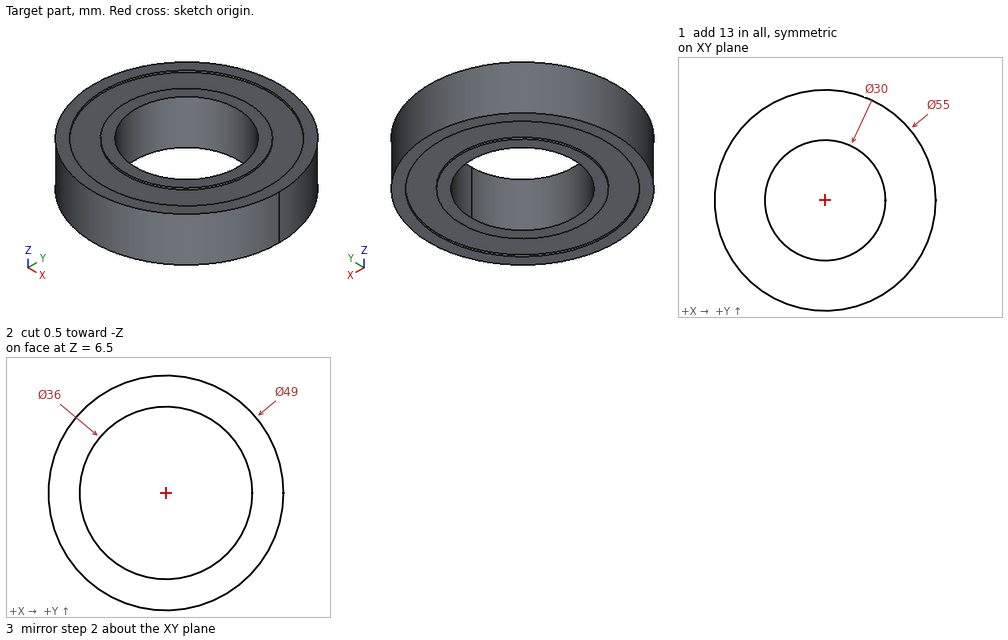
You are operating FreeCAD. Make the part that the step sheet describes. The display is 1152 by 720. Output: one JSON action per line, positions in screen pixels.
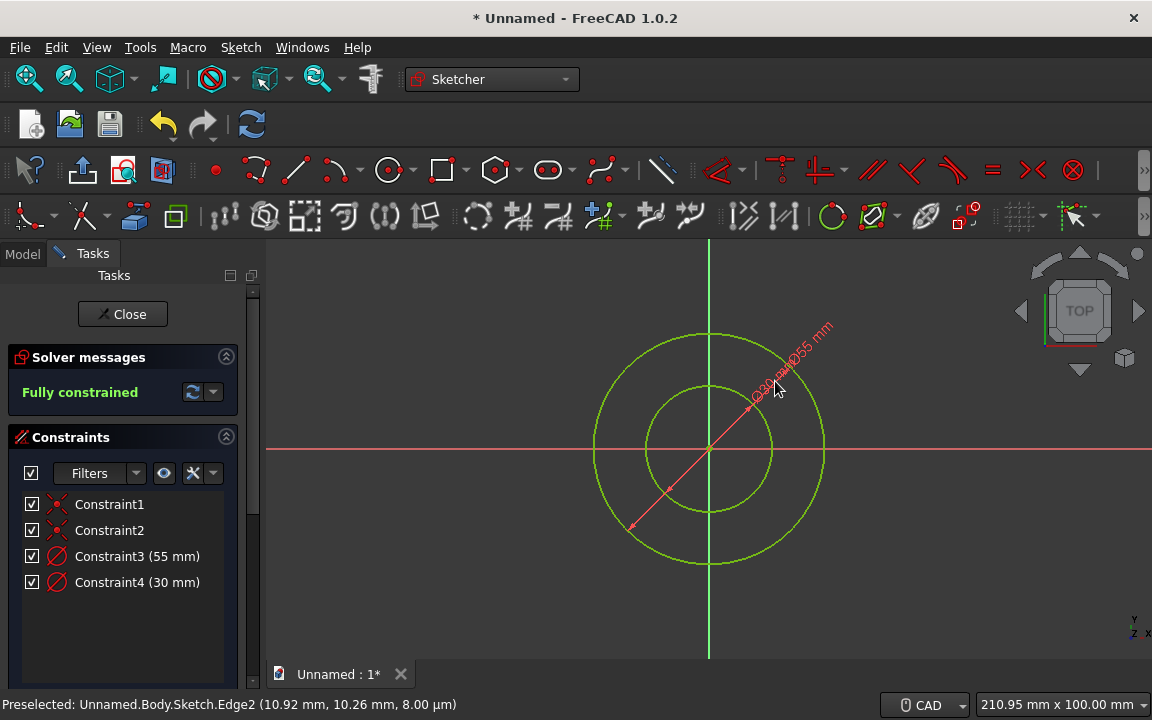
{"action": "left_click", "coordinate": [123, 314]}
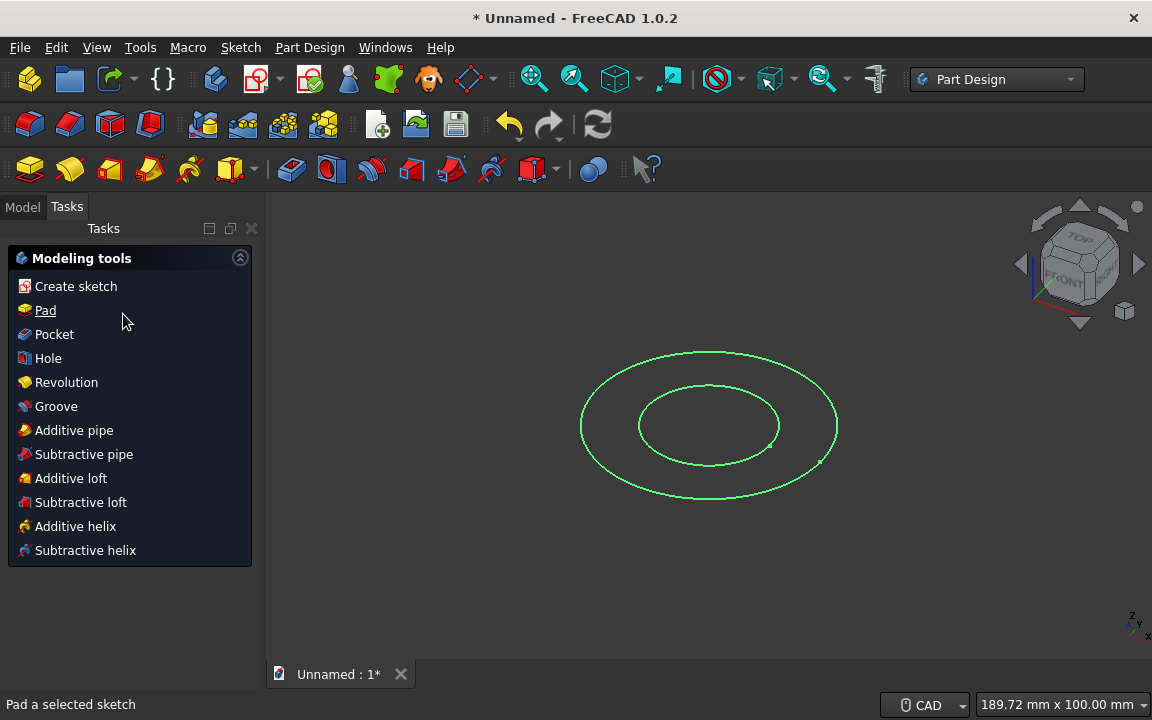
{"action": "left_click", "coordinate": [30, 170]}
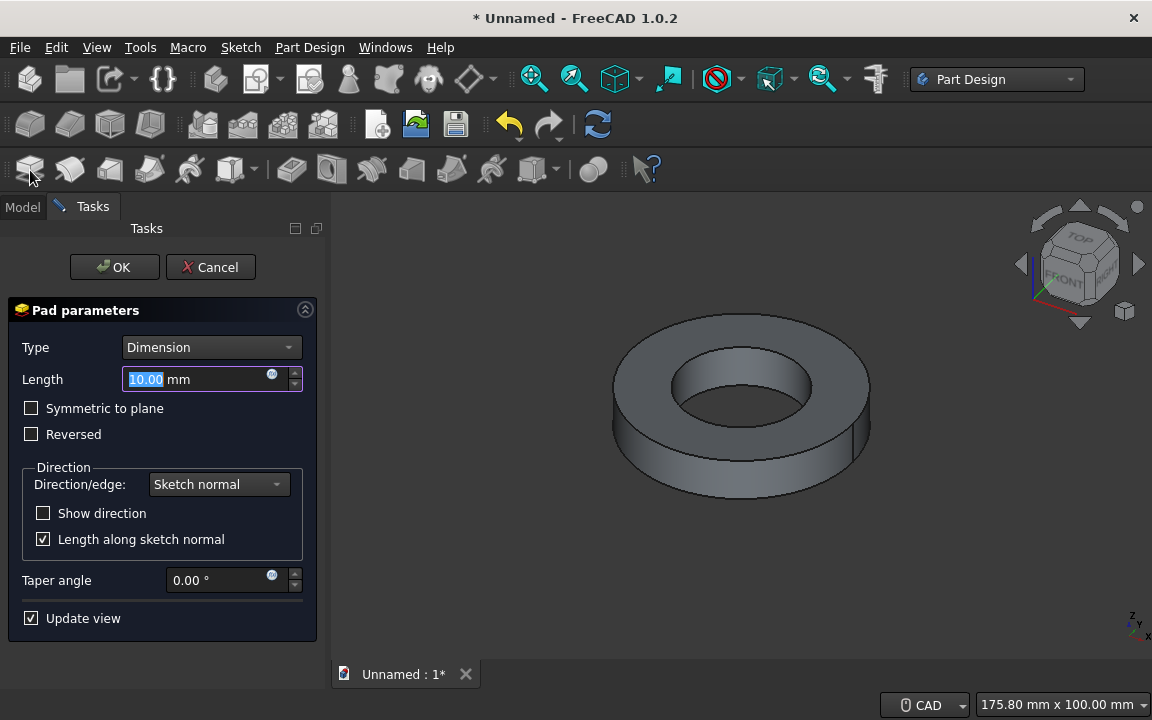
{"action": "type", "text": "13"}
{"action": "key", "text": "Tab"}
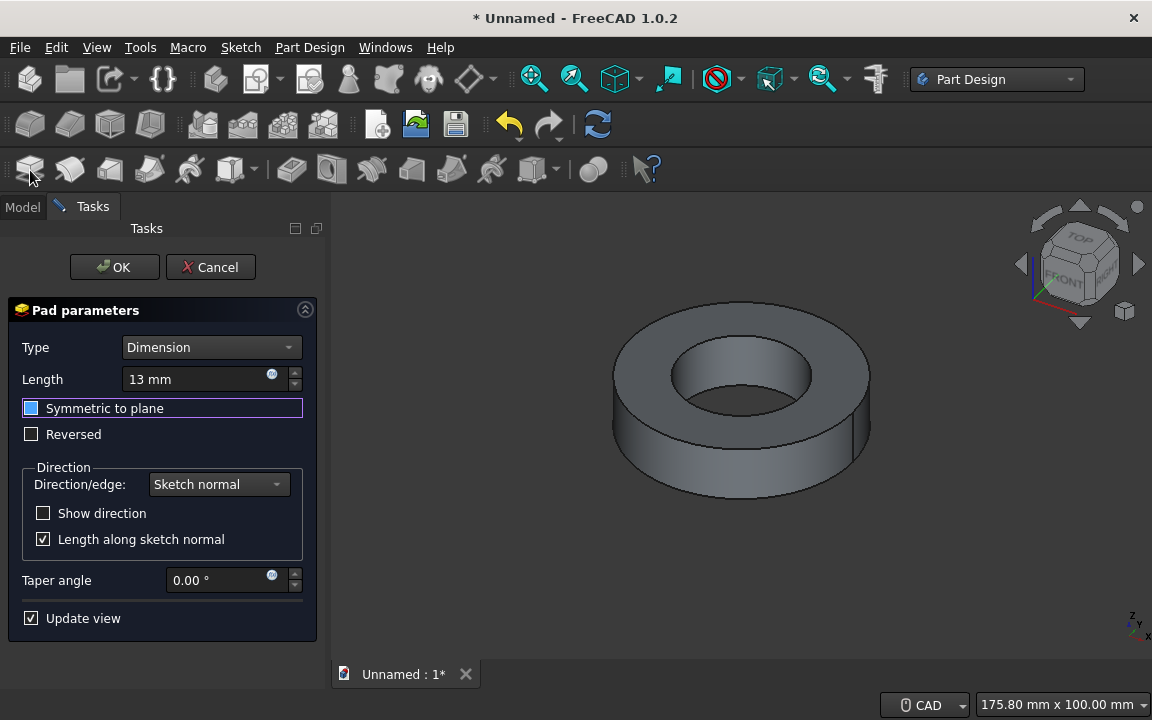
{"action": "left_click", "coordinate": [30, 408]}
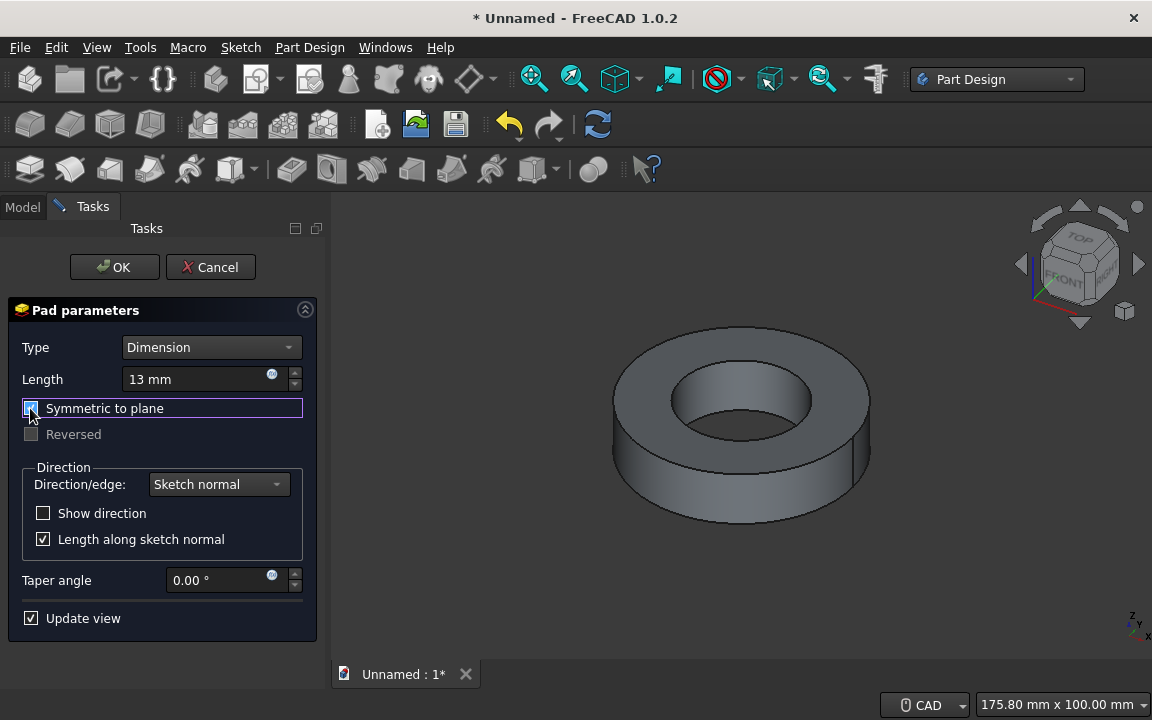
{"action": "left_click", "coordinate": [115, 267]}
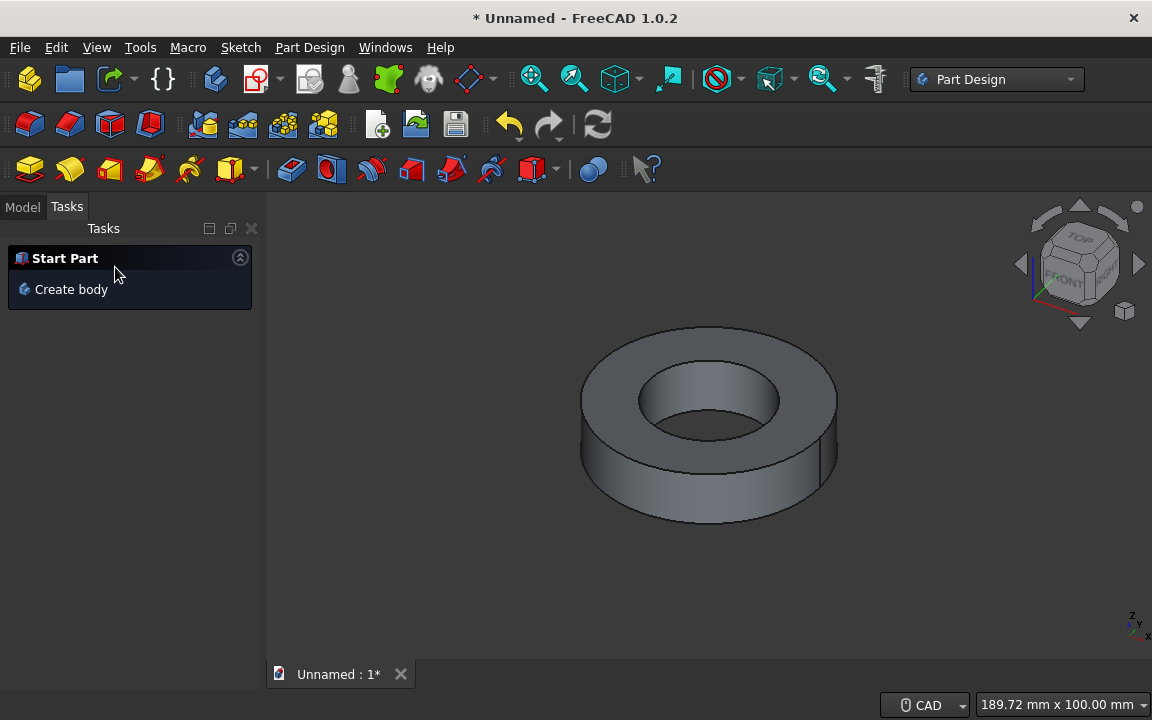
{"action": "left_click", "coordinate": [609, 415]}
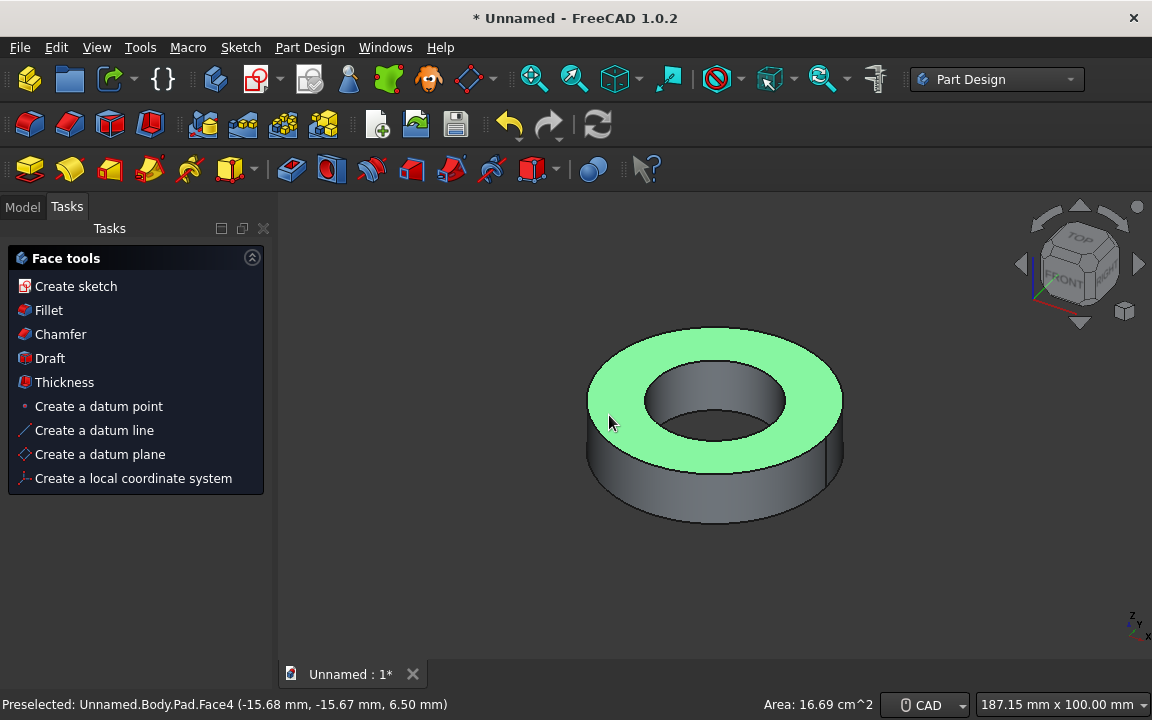
{"action": "left_click", "coordinate": [256, 80]}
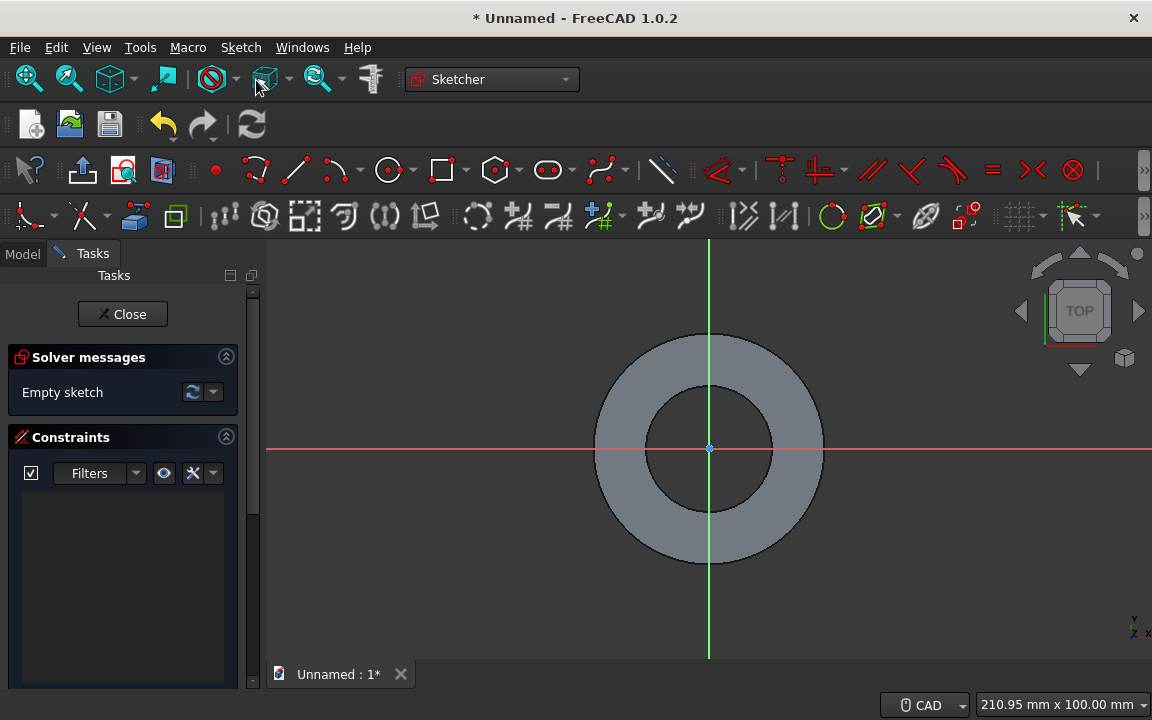
{"action": "left_click", "coordinate": [390, 170]}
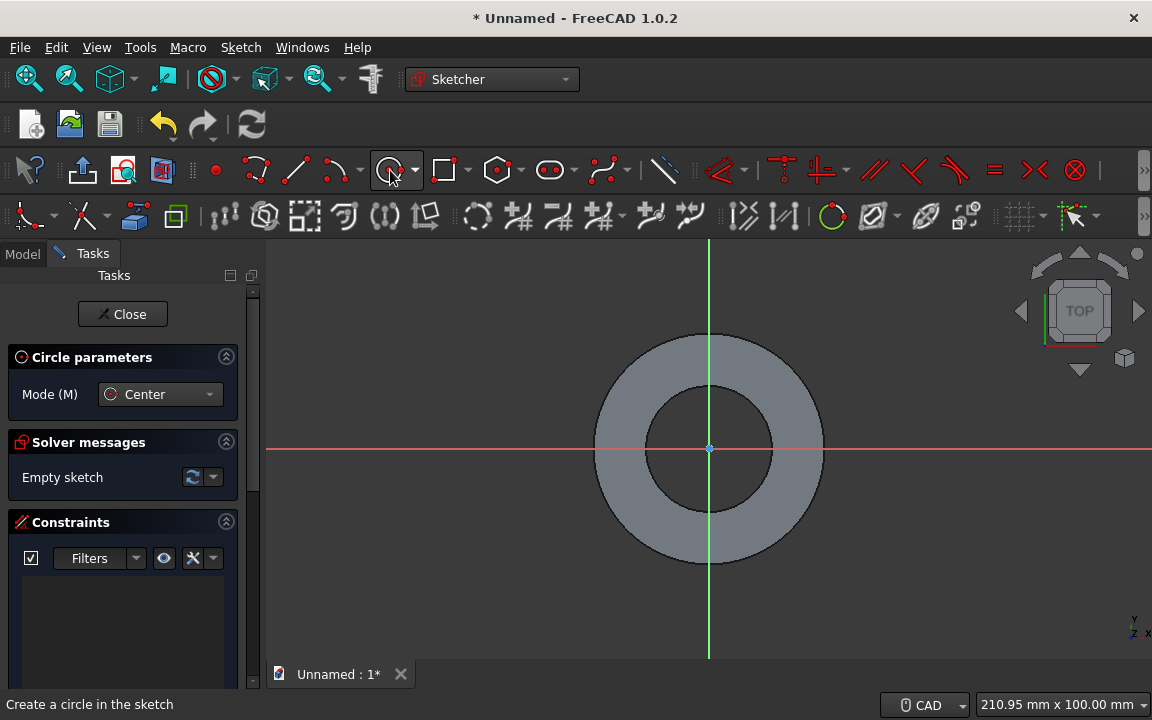
{"action": "left_click", "coordinate": [709, 449]}
{"action": "left_click", "coordinate": [782, 376]}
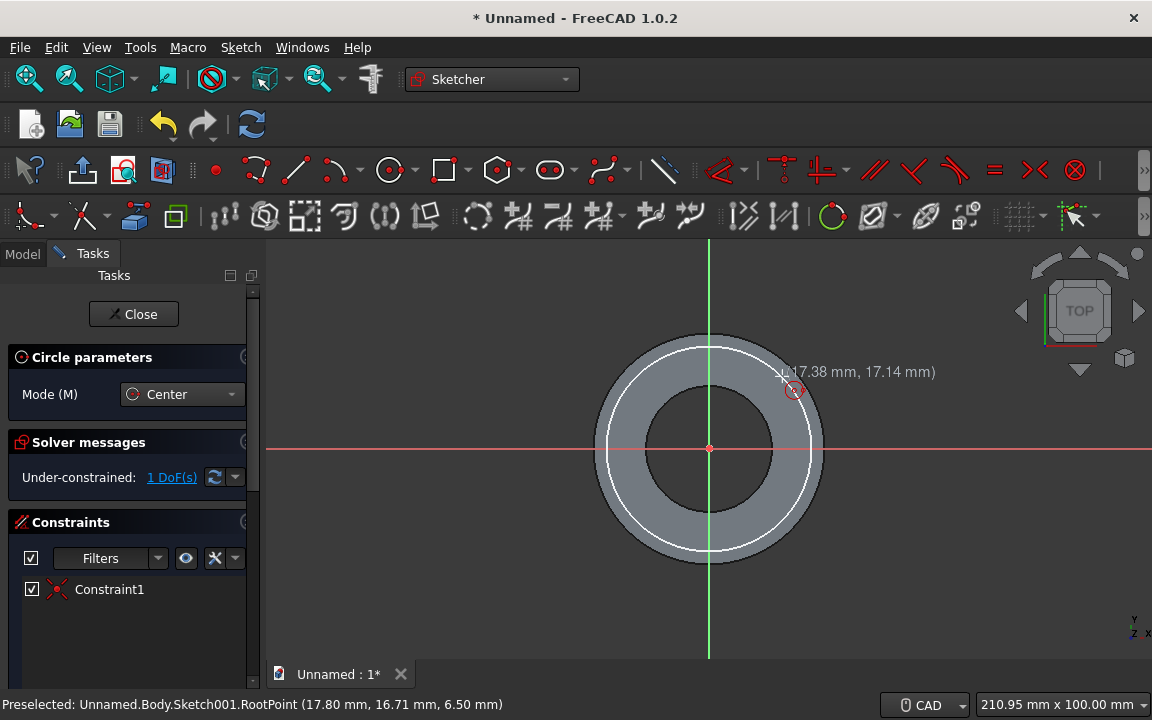
{"action": "left_click", "coordinate": [709, 449]}
{"action": "left_click", "coordinate": [762, 396]}
{"action": "key", "text": "Escape"}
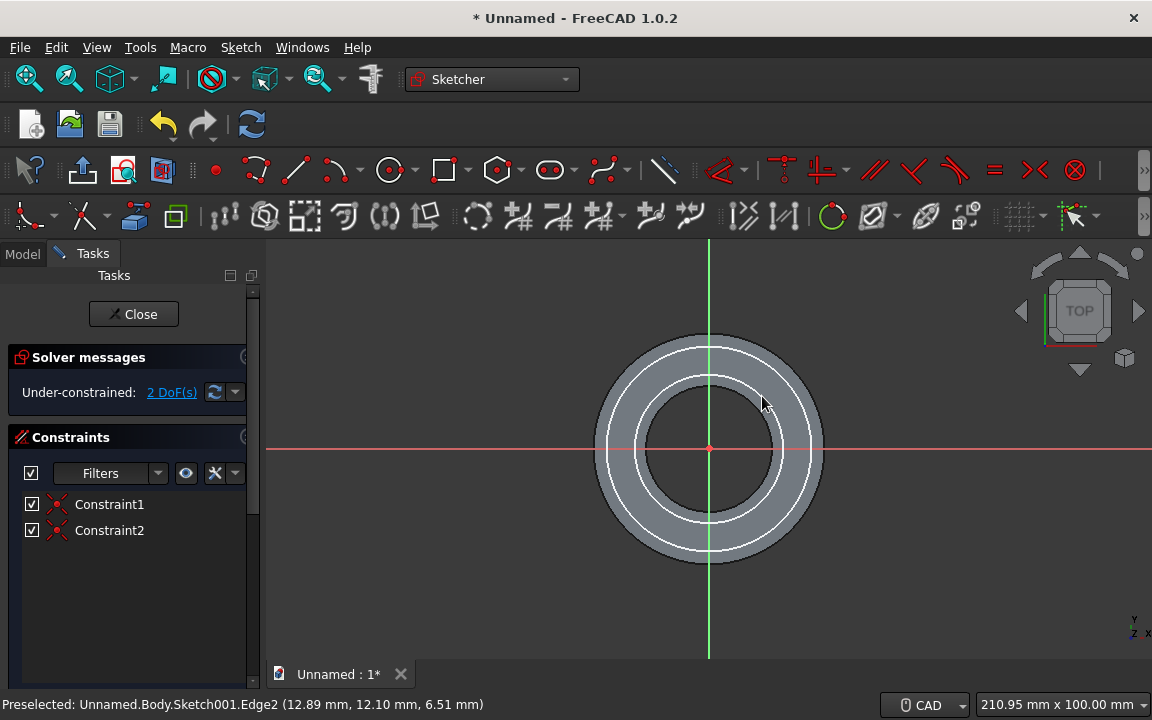
{"action": "left_click", "coordinate": [720, 170]}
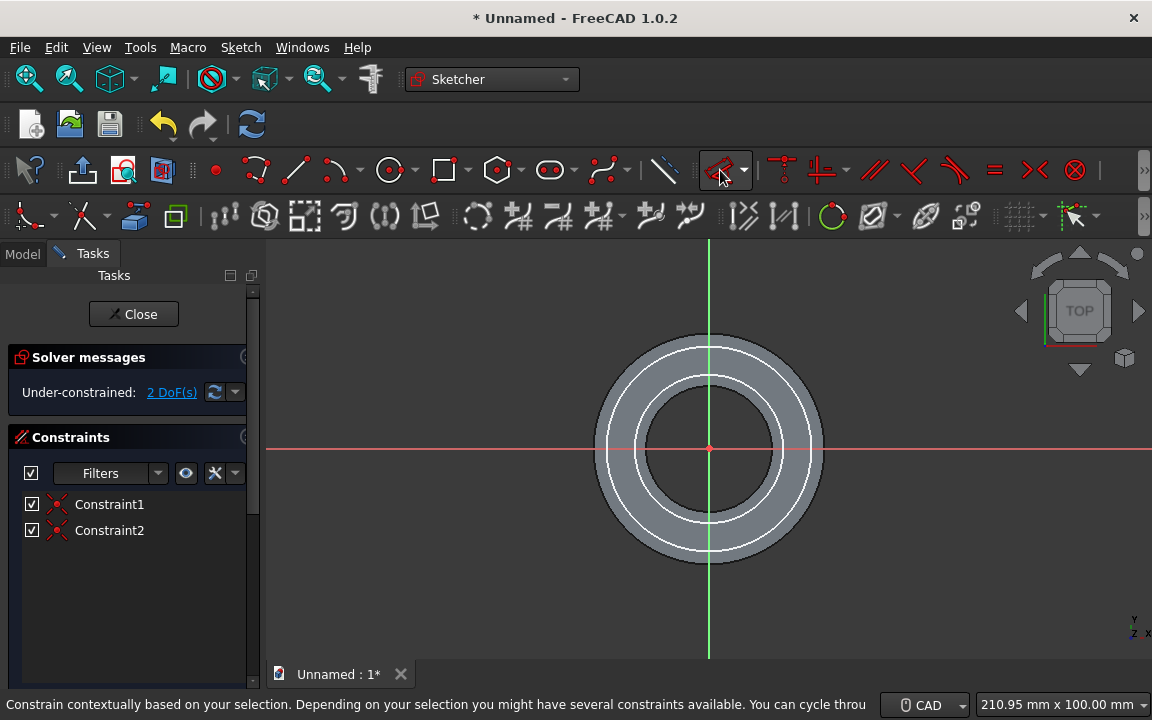
{"action": "left_click", "coordinate": [781, 376]}
{"action": "left_click", "coordinate": [803, 353]}